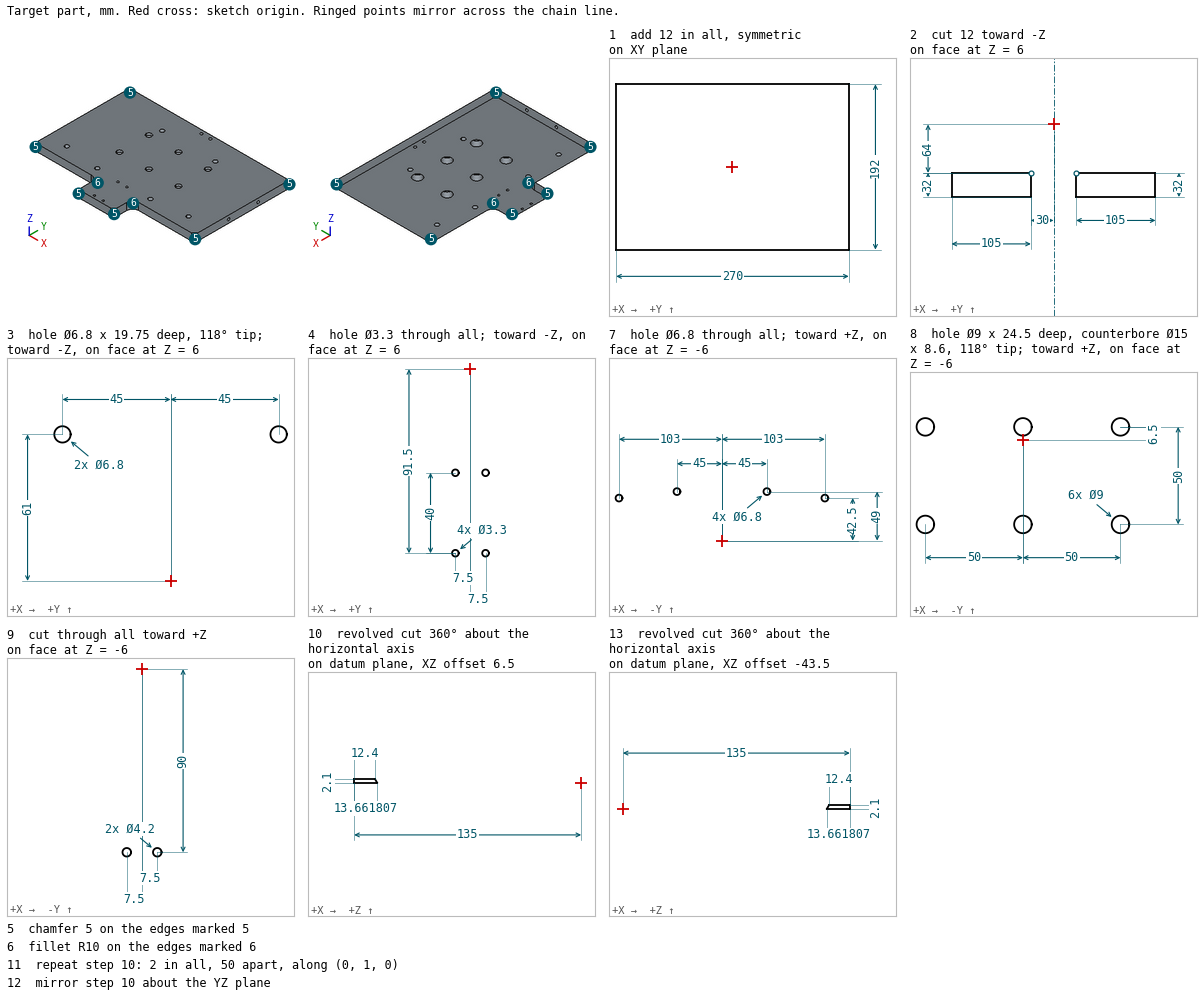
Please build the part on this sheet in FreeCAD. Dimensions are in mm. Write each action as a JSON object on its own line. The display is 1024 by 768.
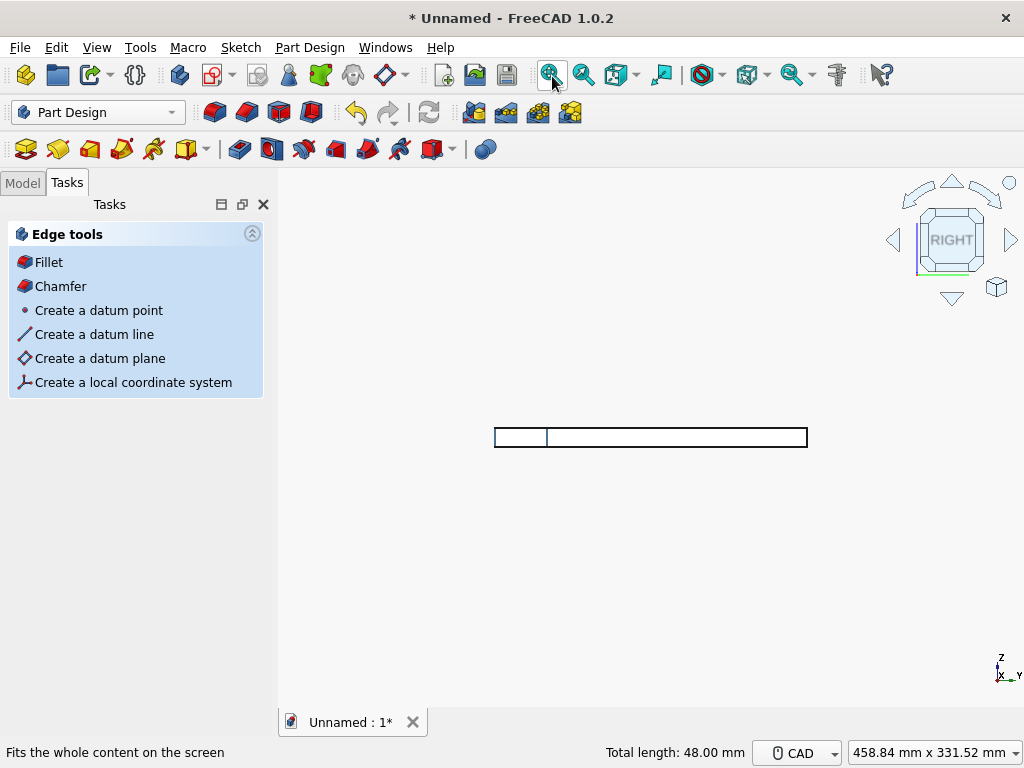
{"action": "left_click", "coordinate": [807, 436], "text": "ctrl"}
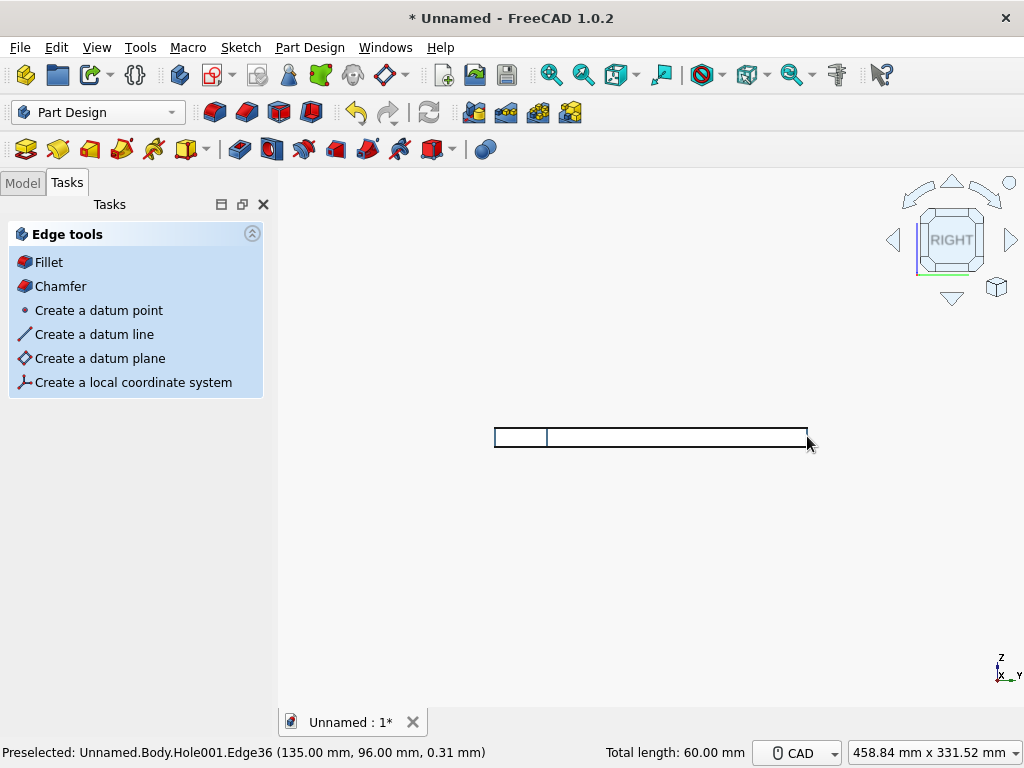
{"action": "scroll", "coordinate": [807, 436], "scroll_direction": "up", "scroll_amount": 4}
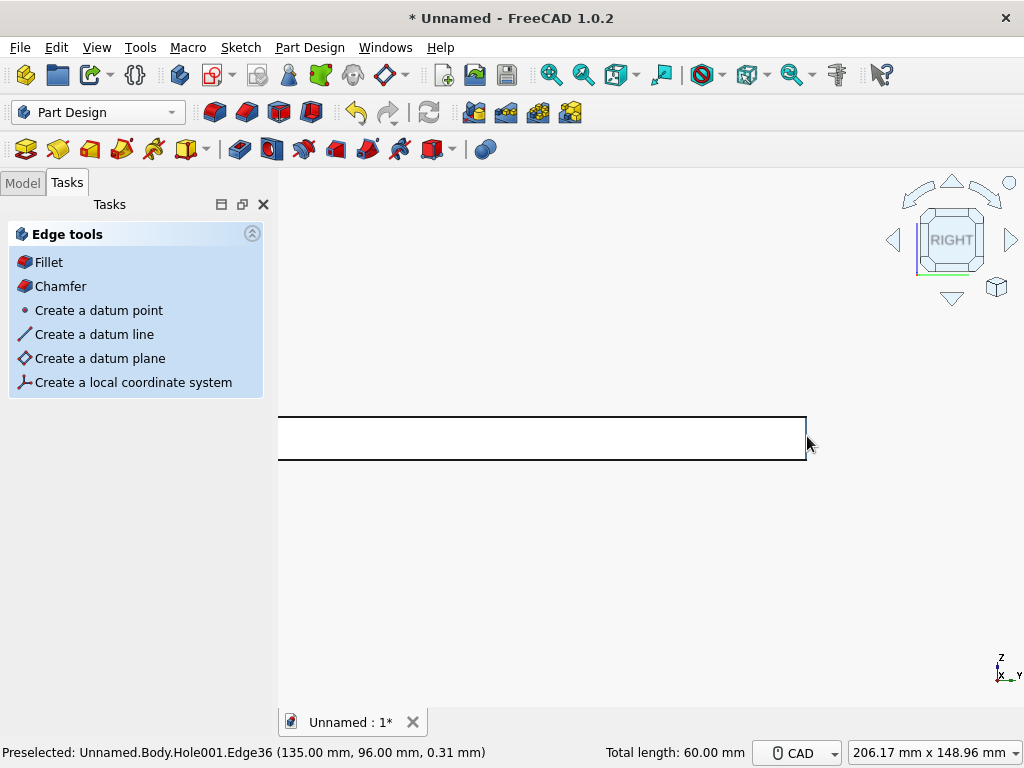
{"action": "key", "text": "v f"}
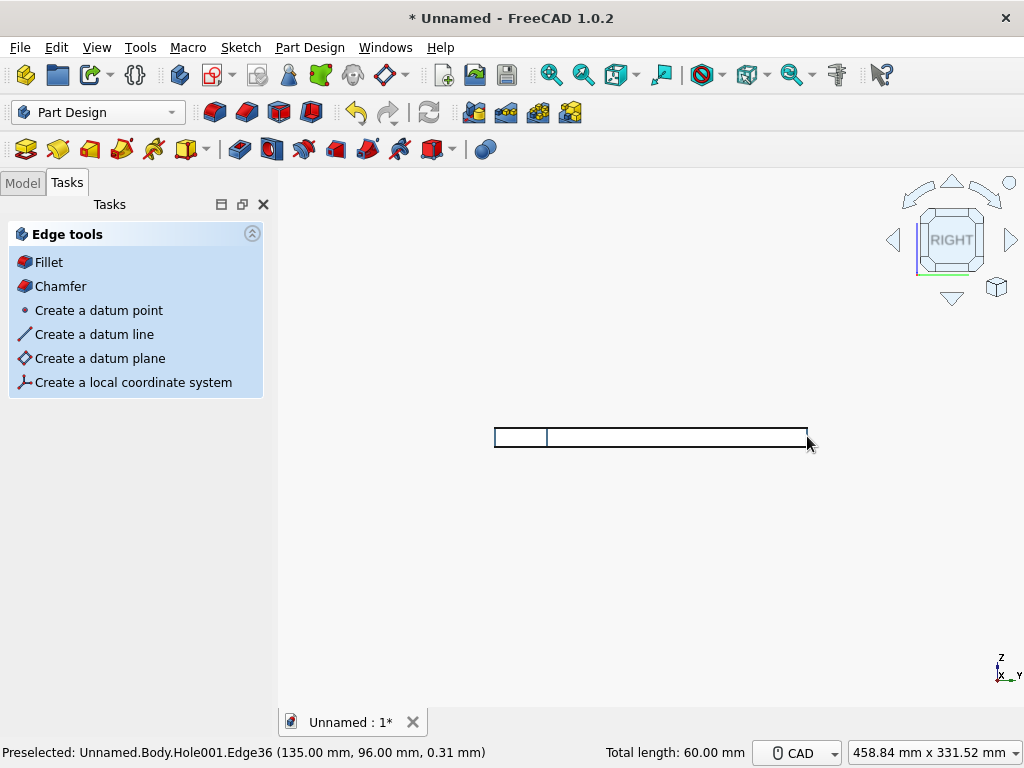
{"action": "key", "text": "5"}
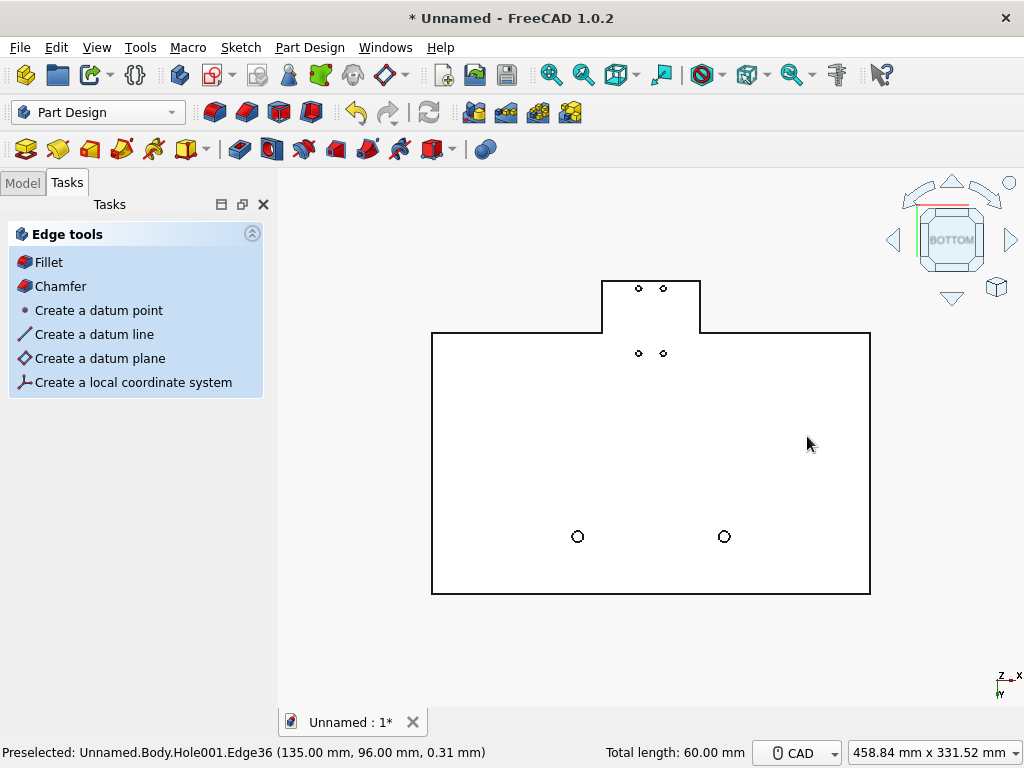
{"action": "scroll", "coordinate": [432, 593], "scroll_direction": "up", "scroll_amount": 4}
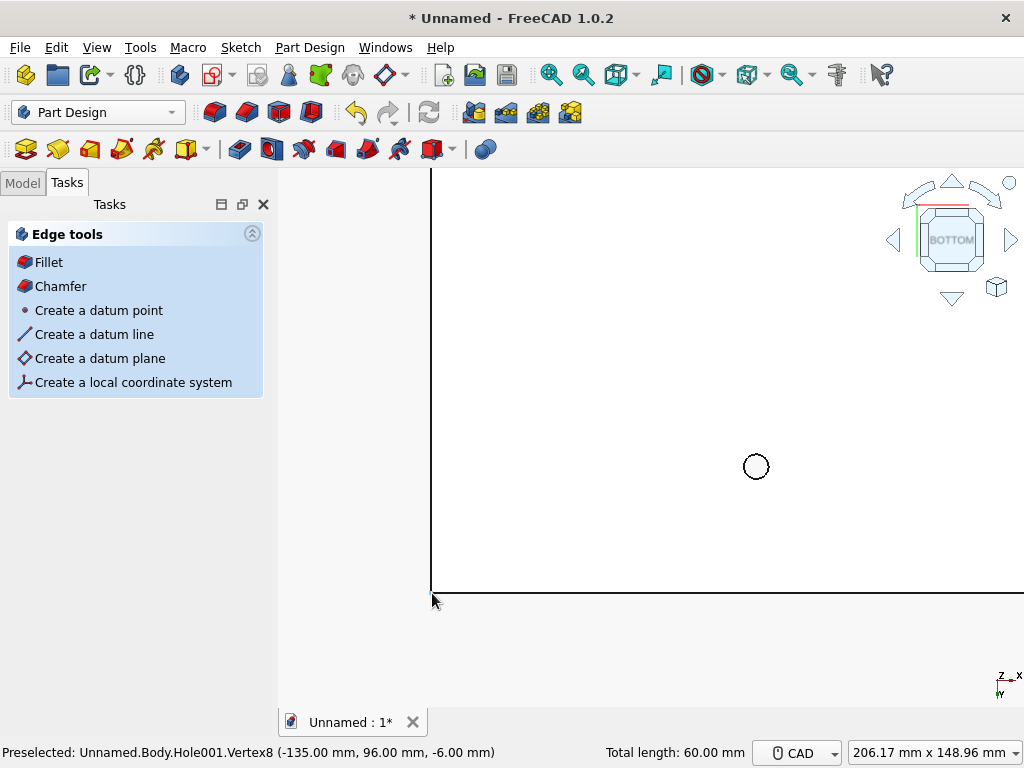
{"action": "key", "text": "v f"}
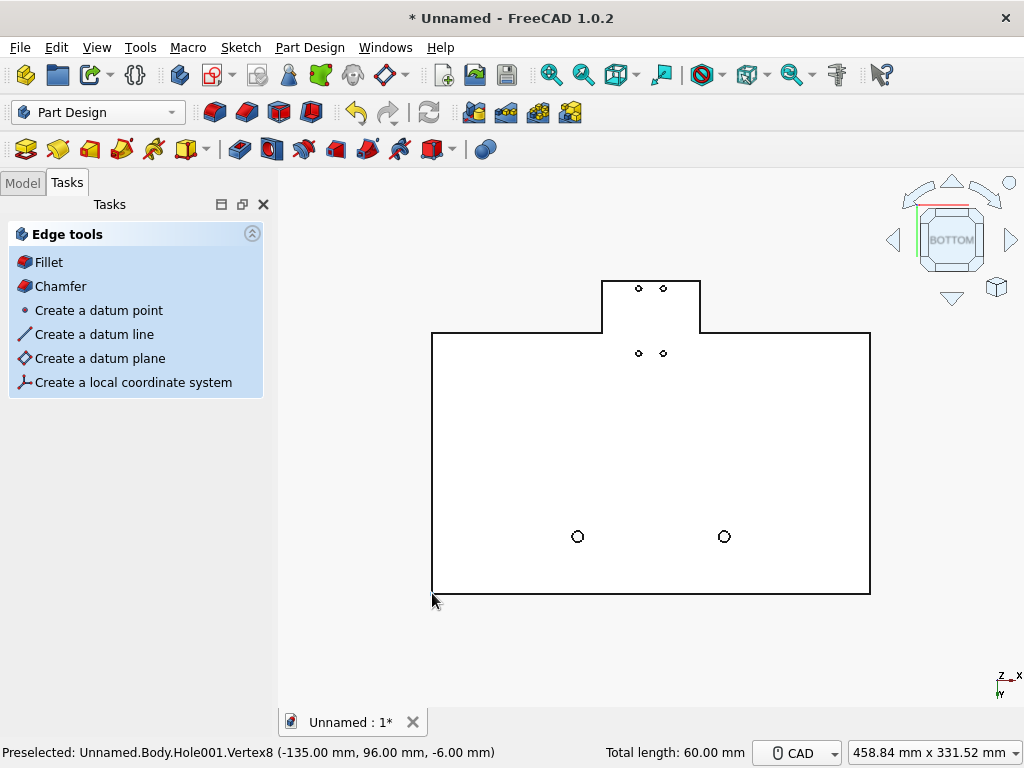
{"action": "key", "text": "4"}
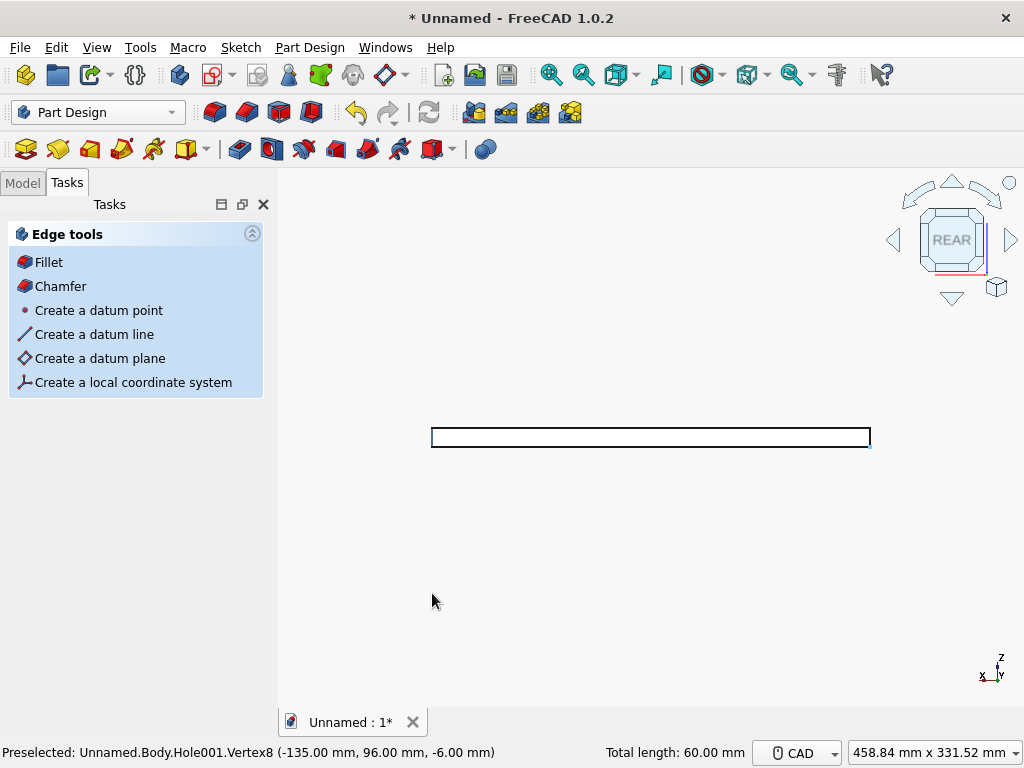
{"action": "left_click", "coordinate": [870, 436], "text": "ctrl"}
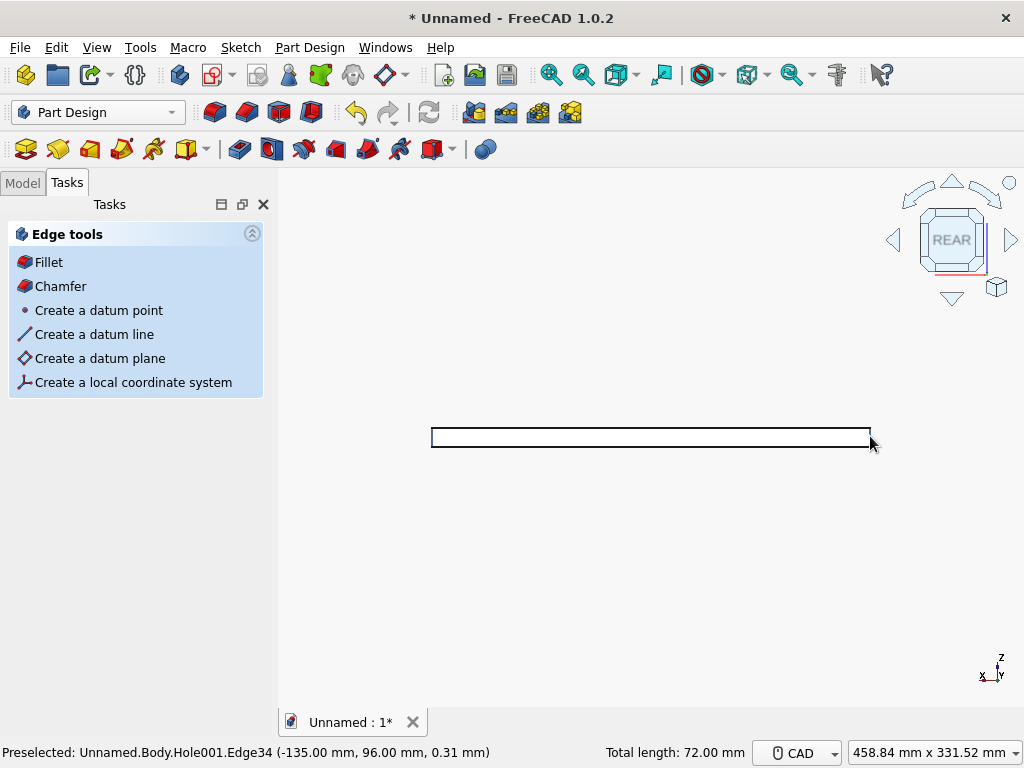
{"action": "left_click", "coordinate": [248, 112]}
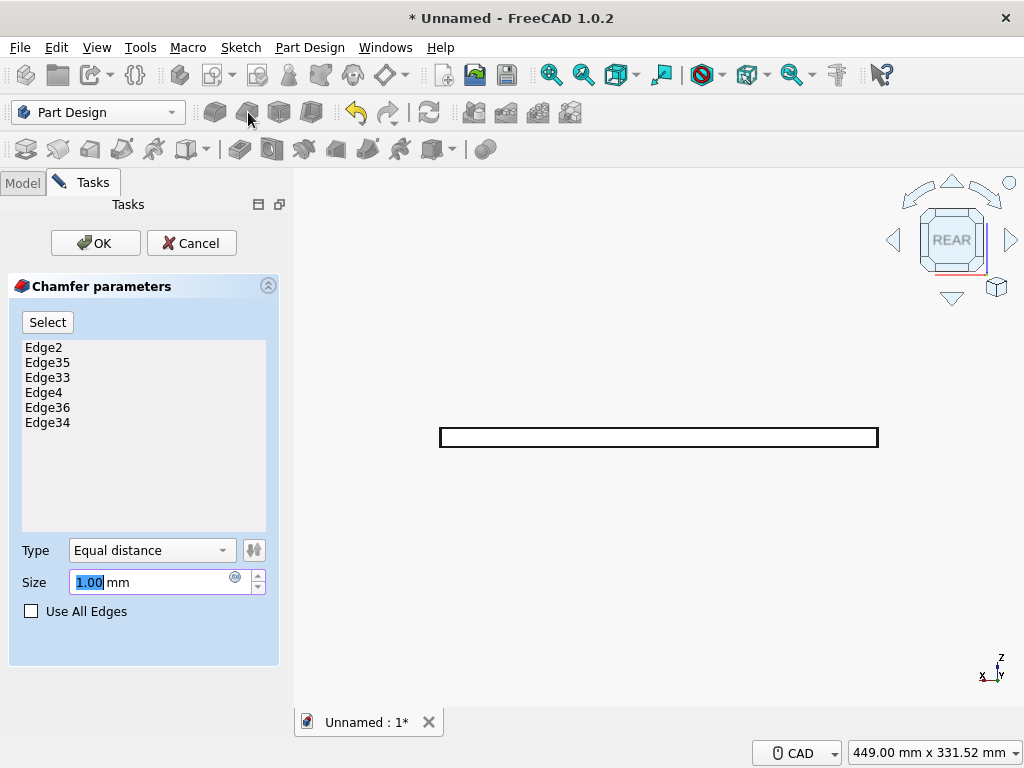
{"action": "type", "text": "5"}
{"action": "key", "text": "Tab"}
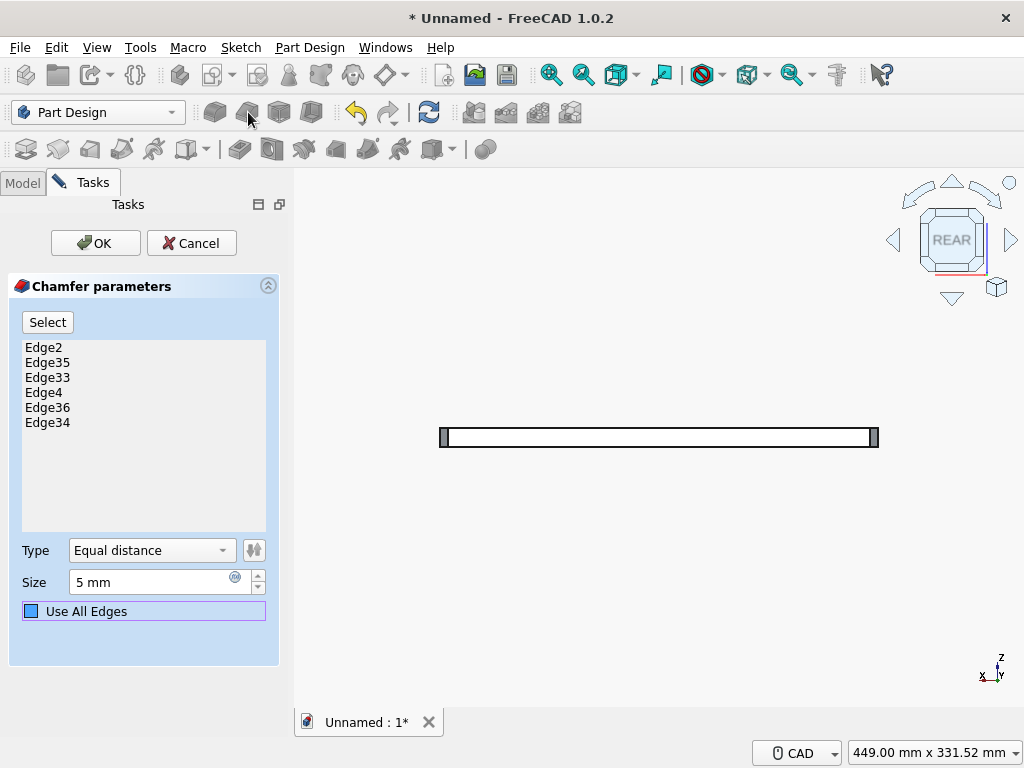
{"action": "left_click", "coordinate": [96, 243]}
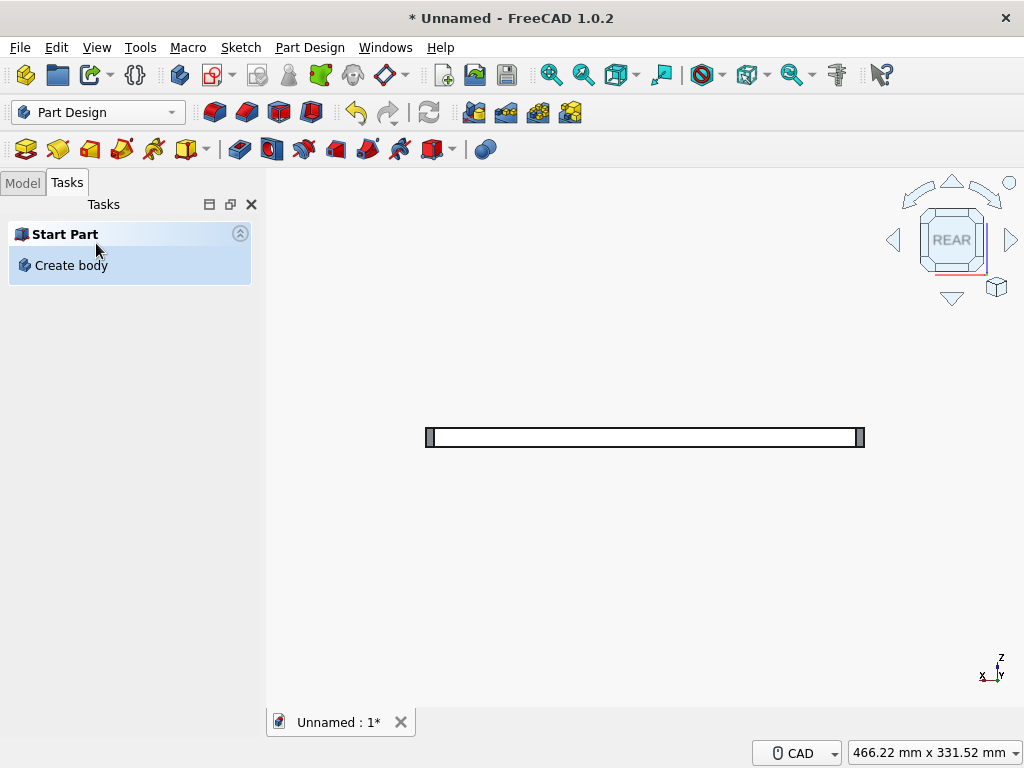
{"action": "scroll", "coordinate": [694, 436], "scroll_direction": "up", "scroll_amount": 4}